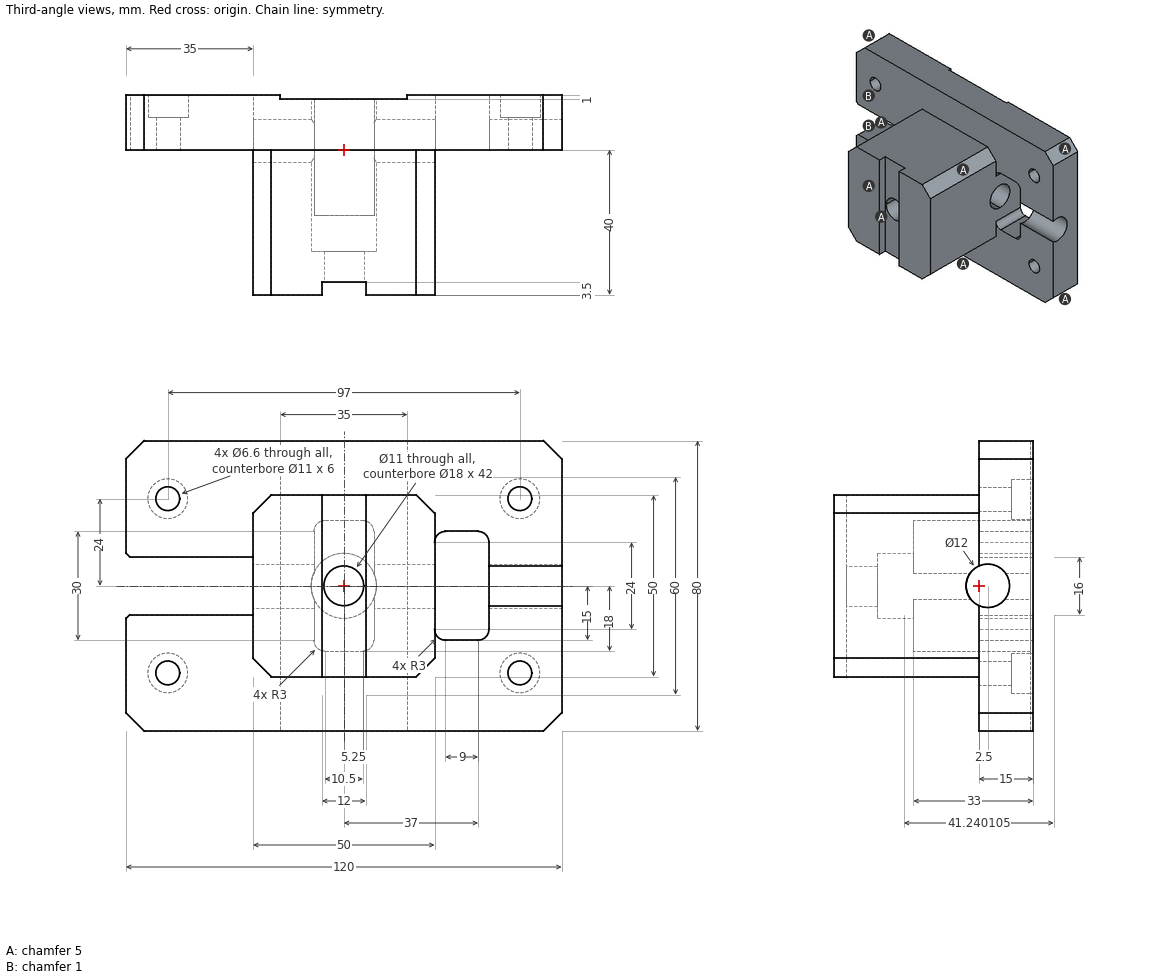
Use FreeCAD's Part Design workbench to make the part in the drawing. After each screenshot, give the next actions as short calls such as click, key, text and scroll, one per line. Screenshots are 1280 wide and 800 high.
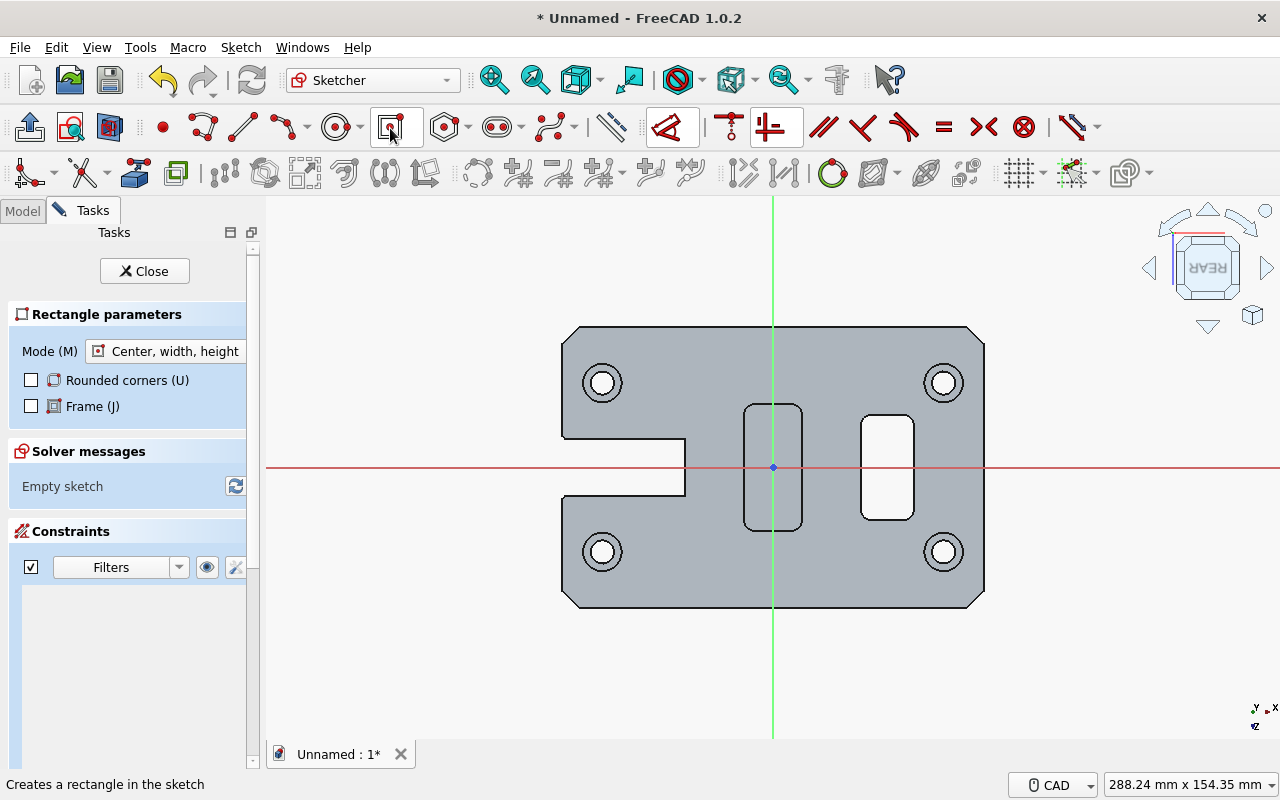
click(773, 467)
click(835, 327)
key(Escape)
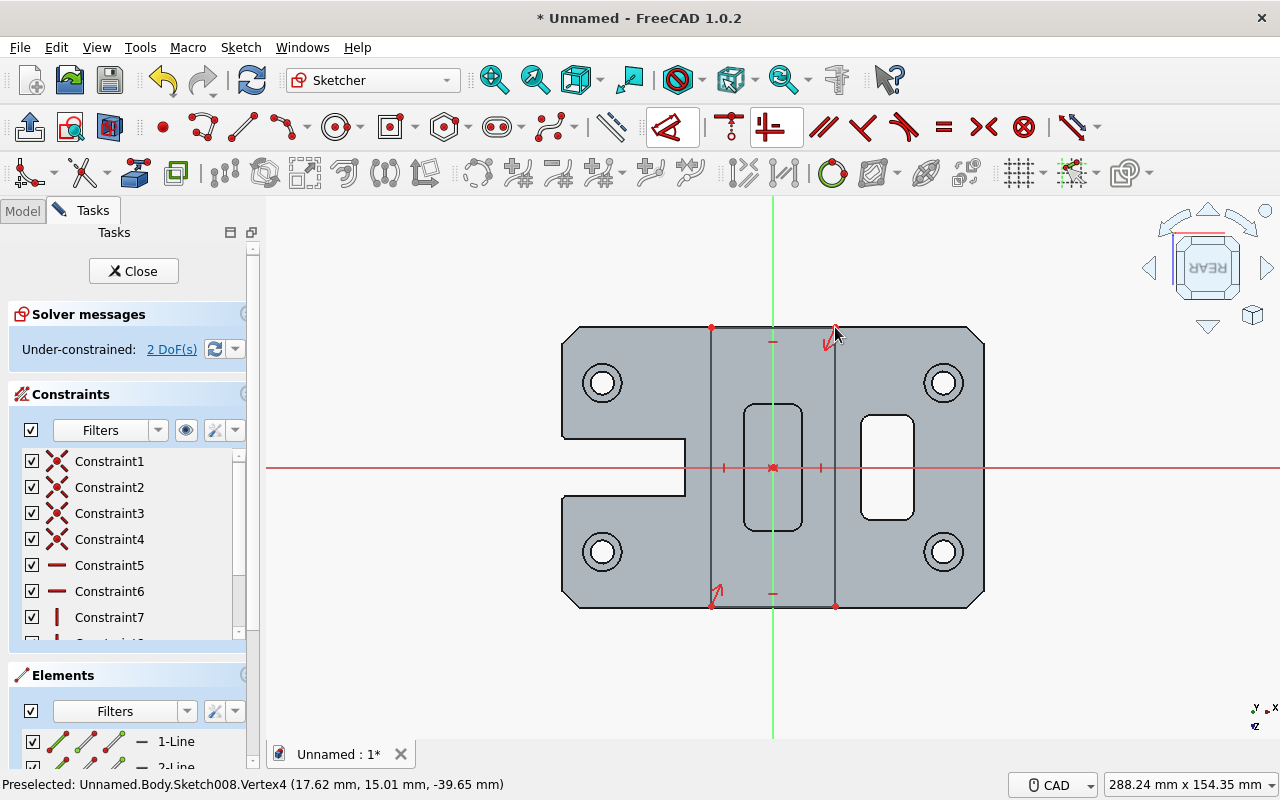
click(748, 607)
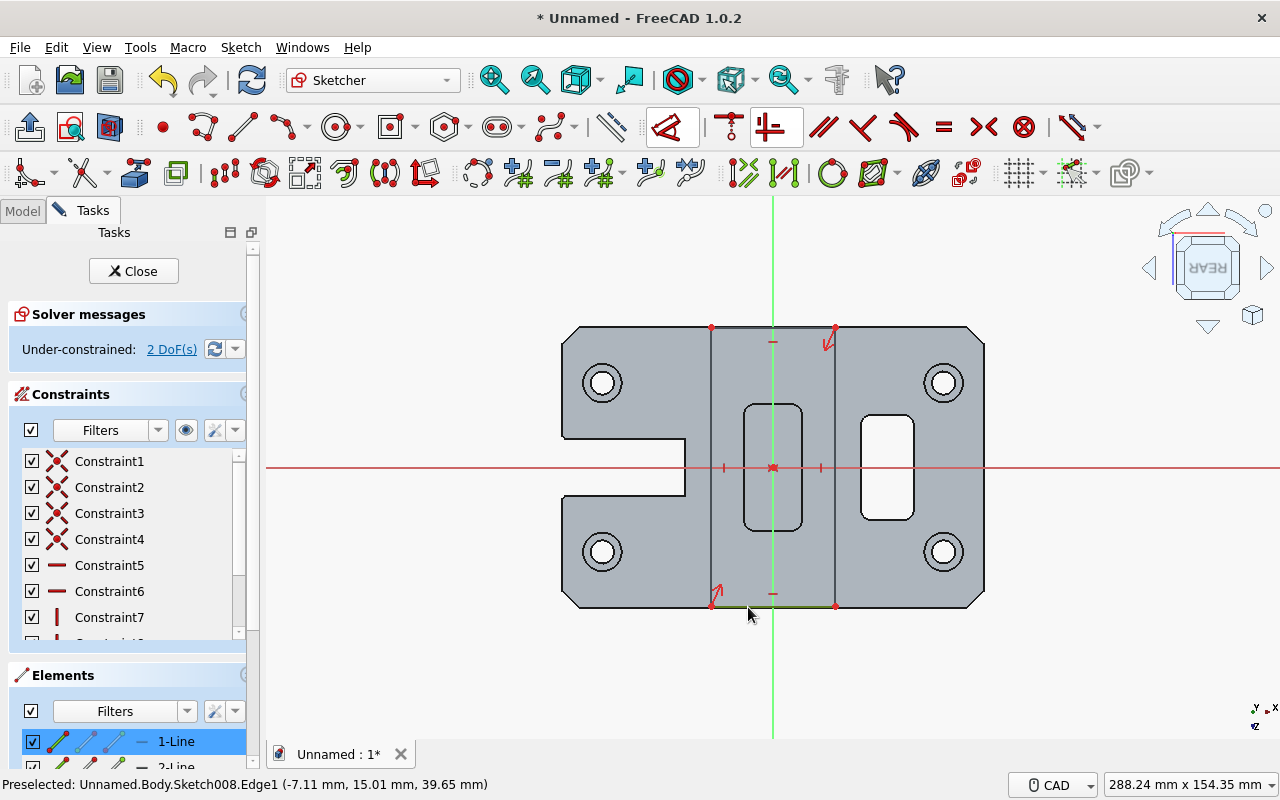
key(l)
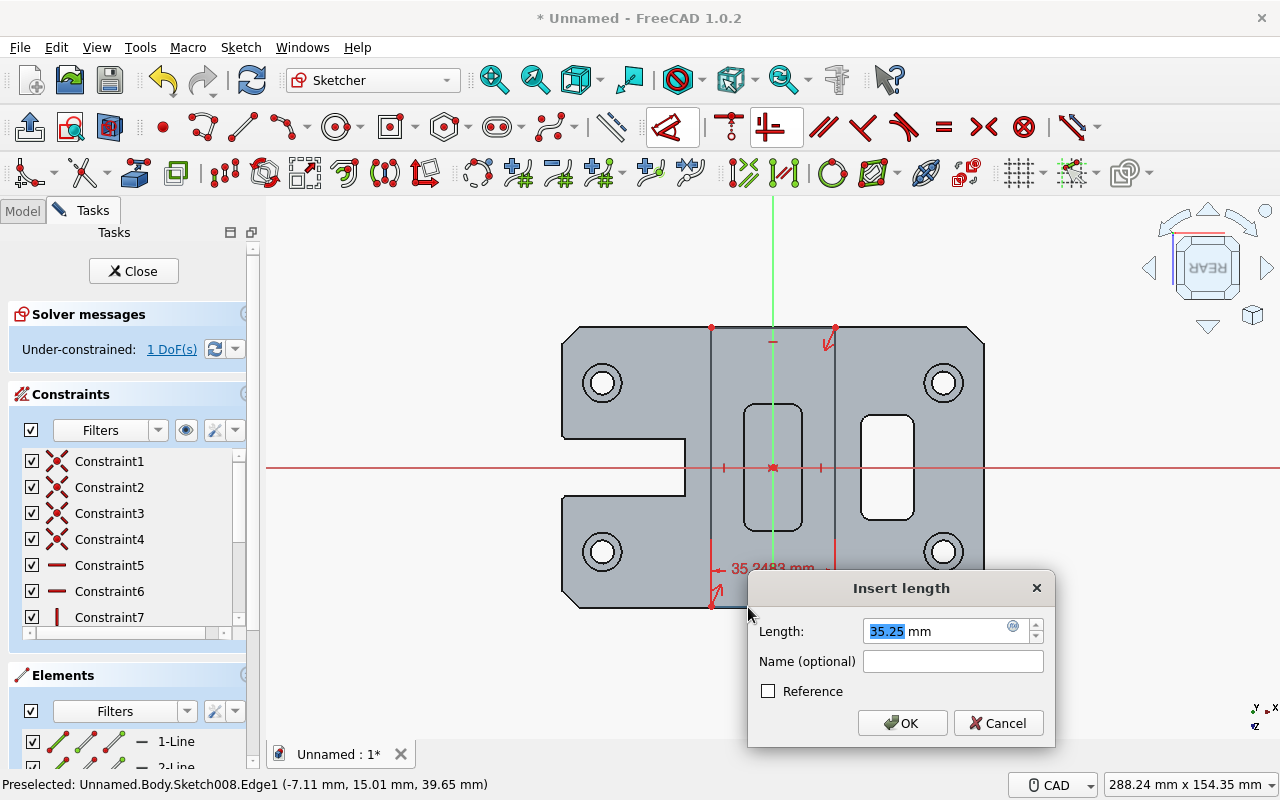
text(35)
key(Return)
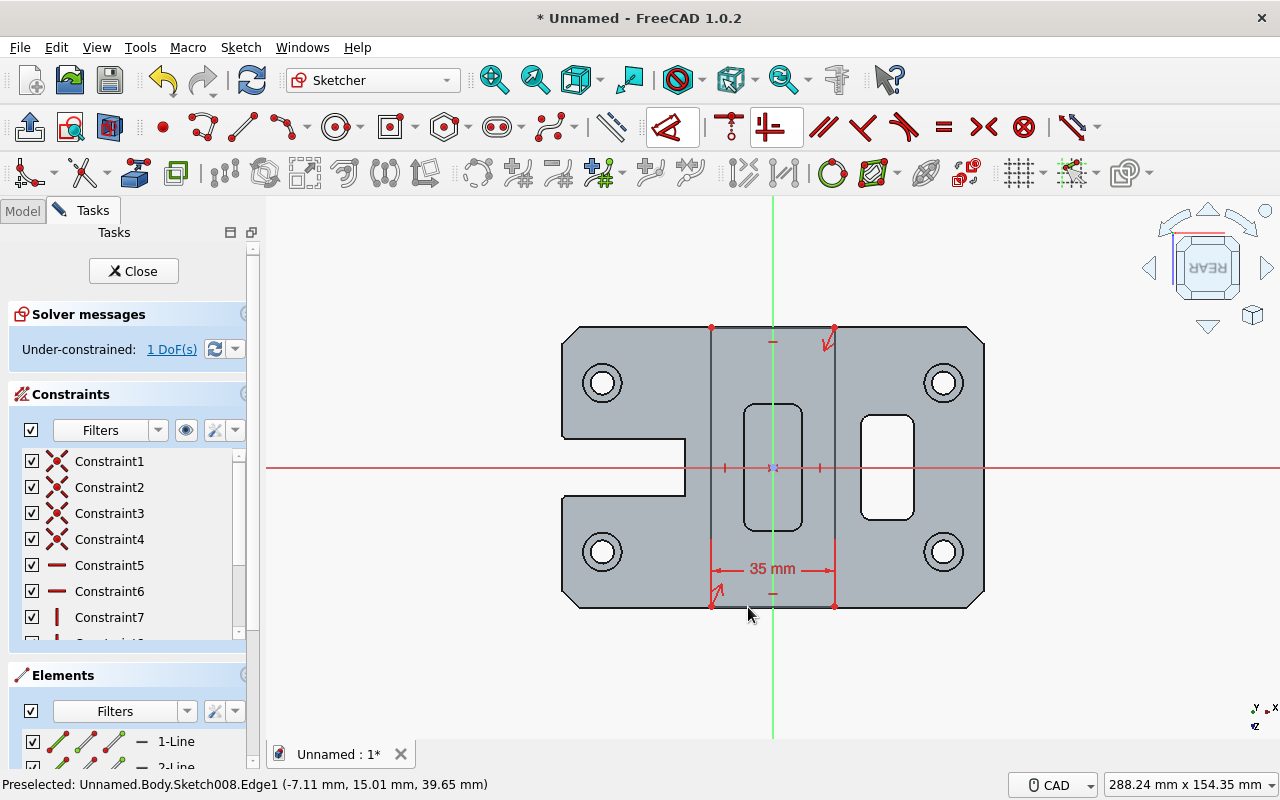
click(835, 523)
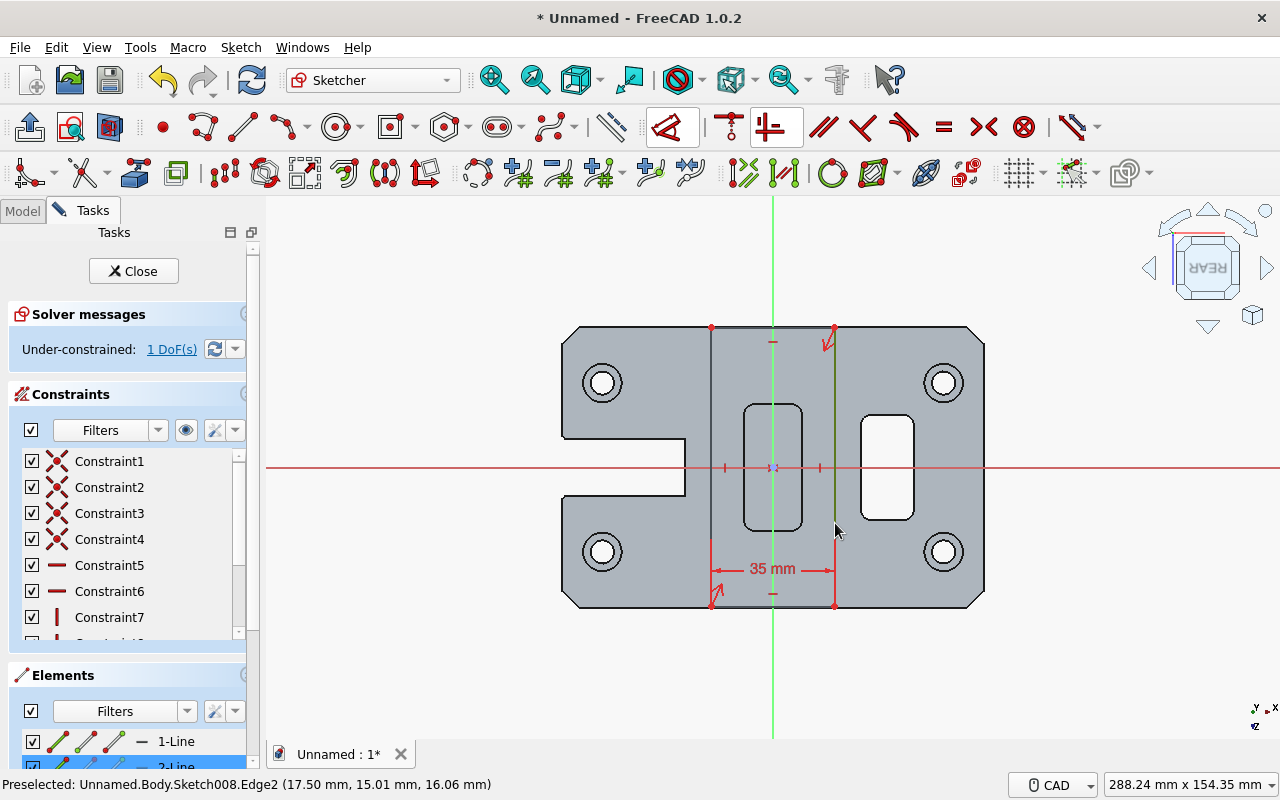
key(i)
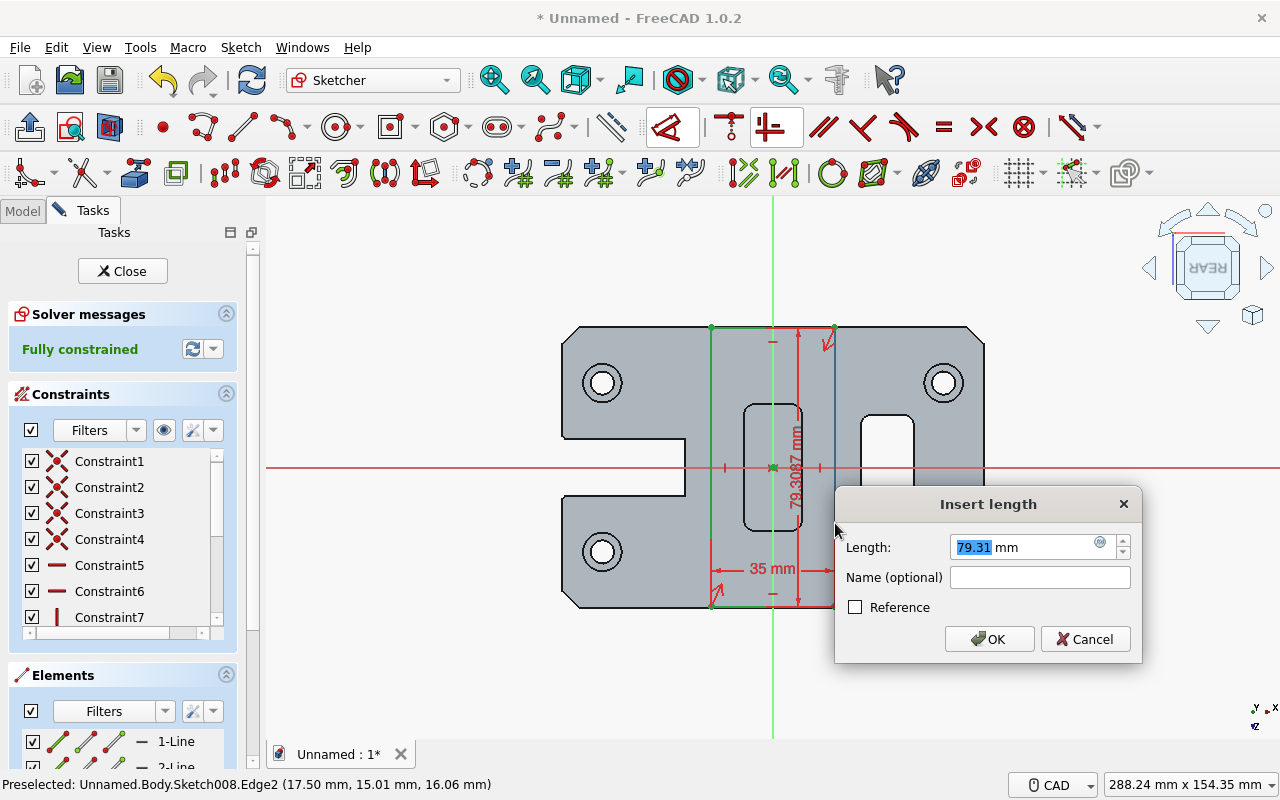
text(80)
key(Return)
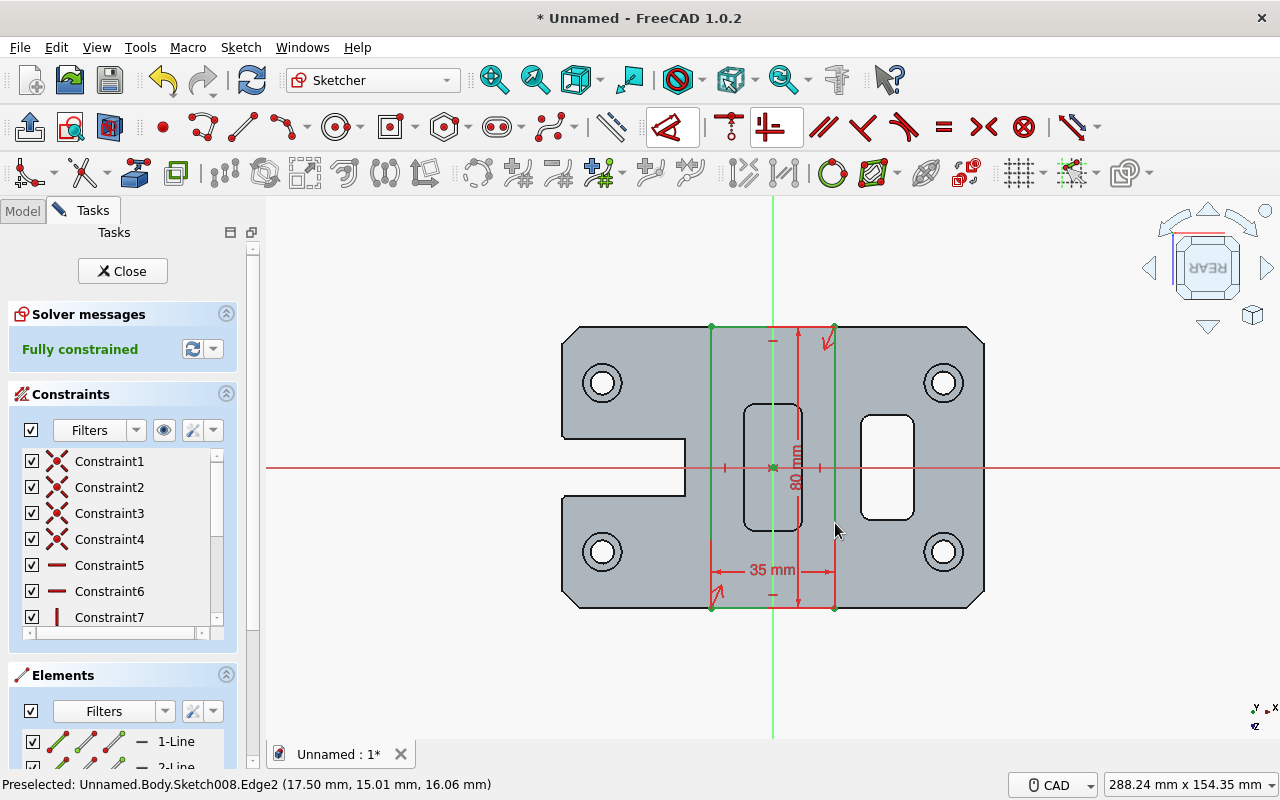
click(123, 271)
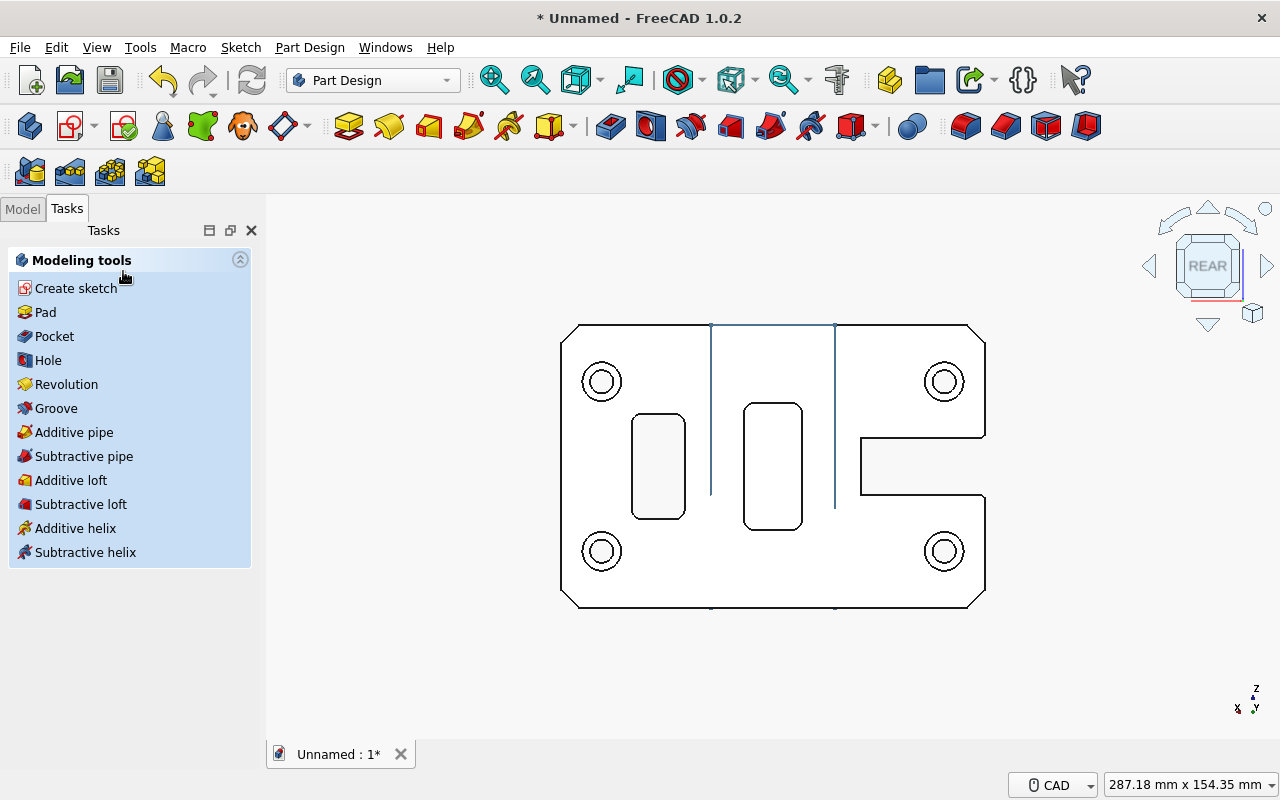
click(612, 126)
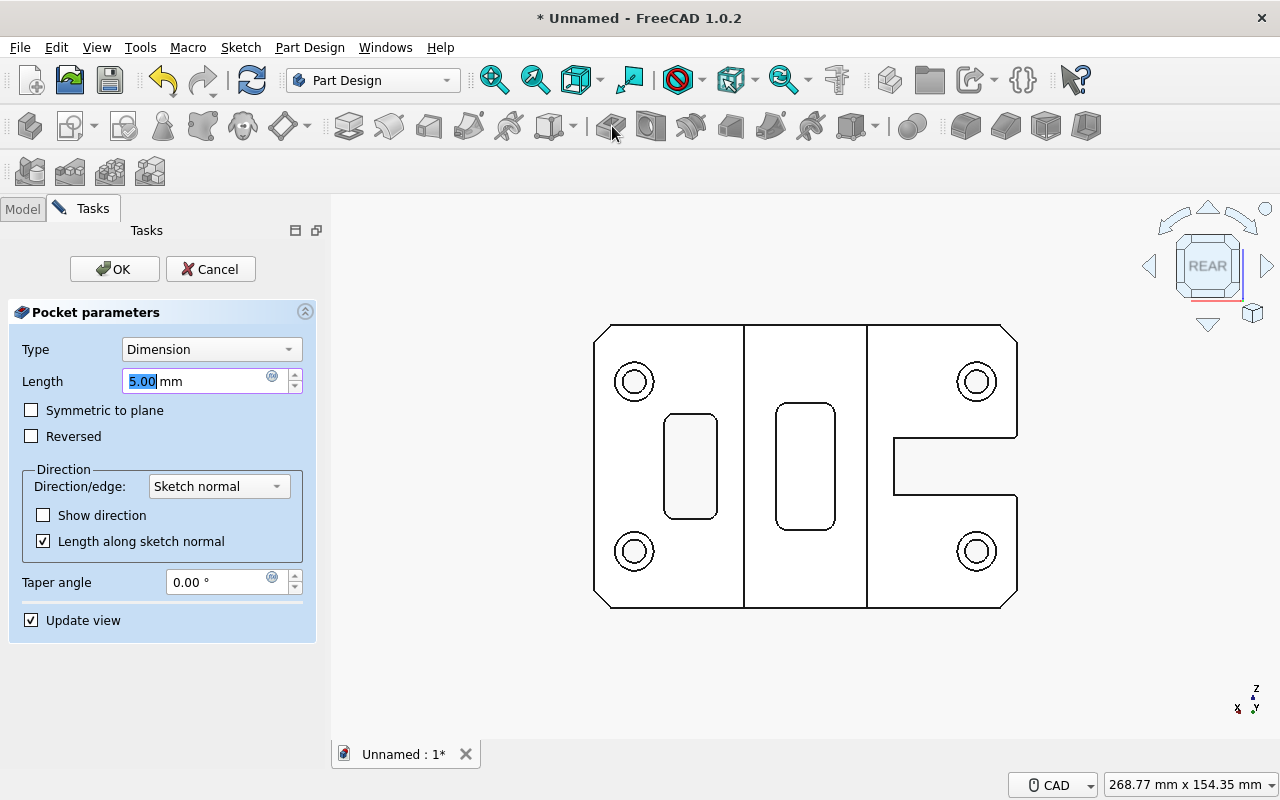
text(1)
key(Tab)